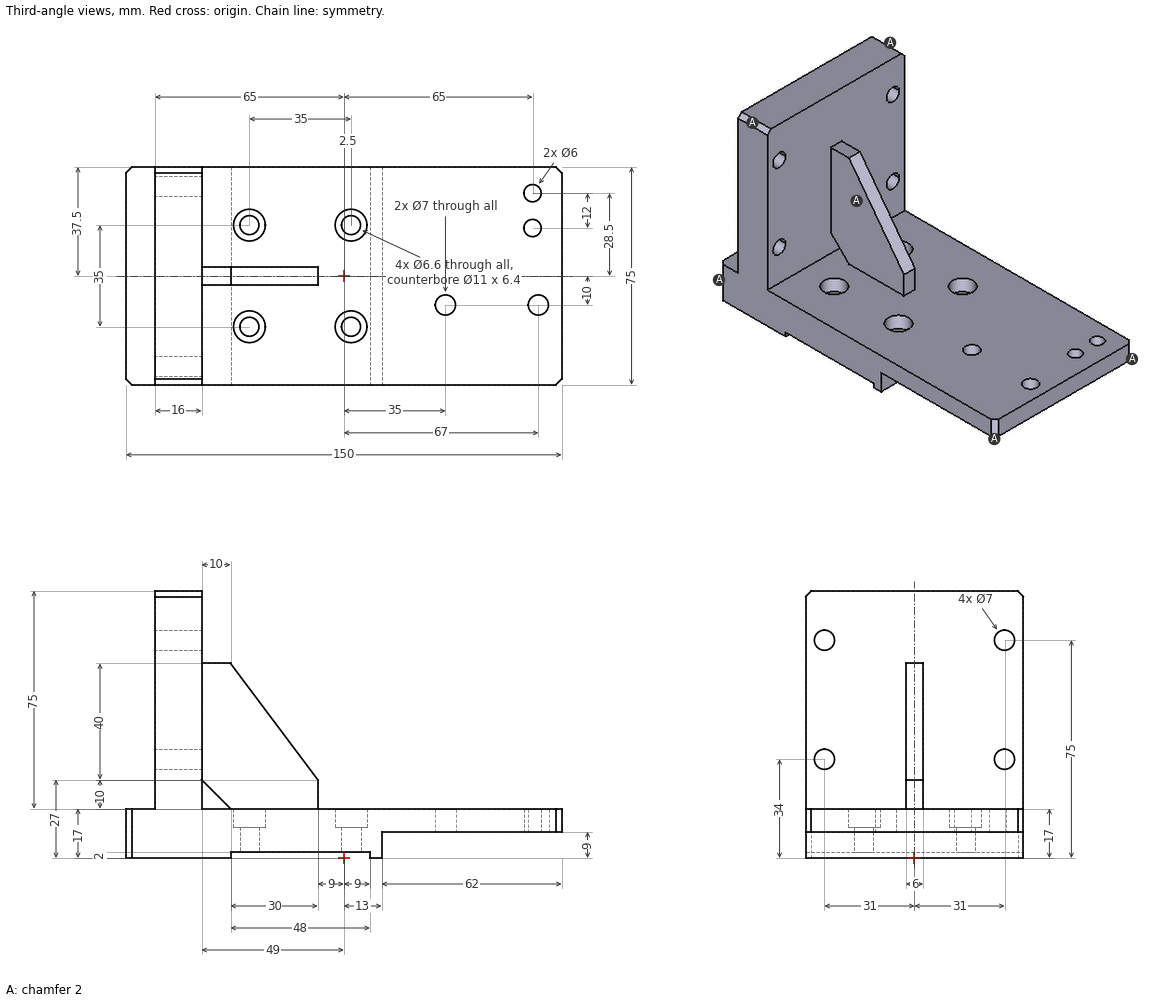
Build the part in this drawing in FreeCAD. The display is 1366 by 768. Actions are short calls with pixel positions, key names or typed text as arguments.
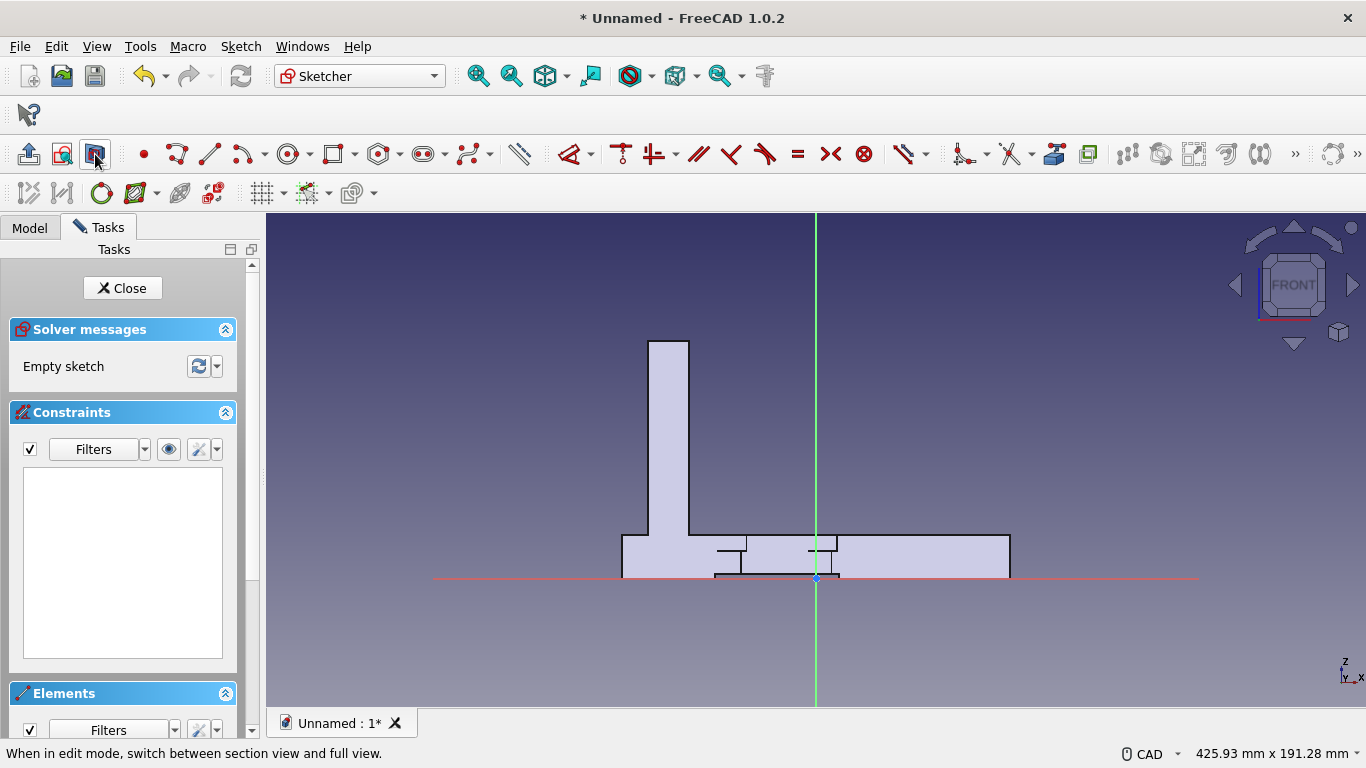
scroll(759, 532, up, 3)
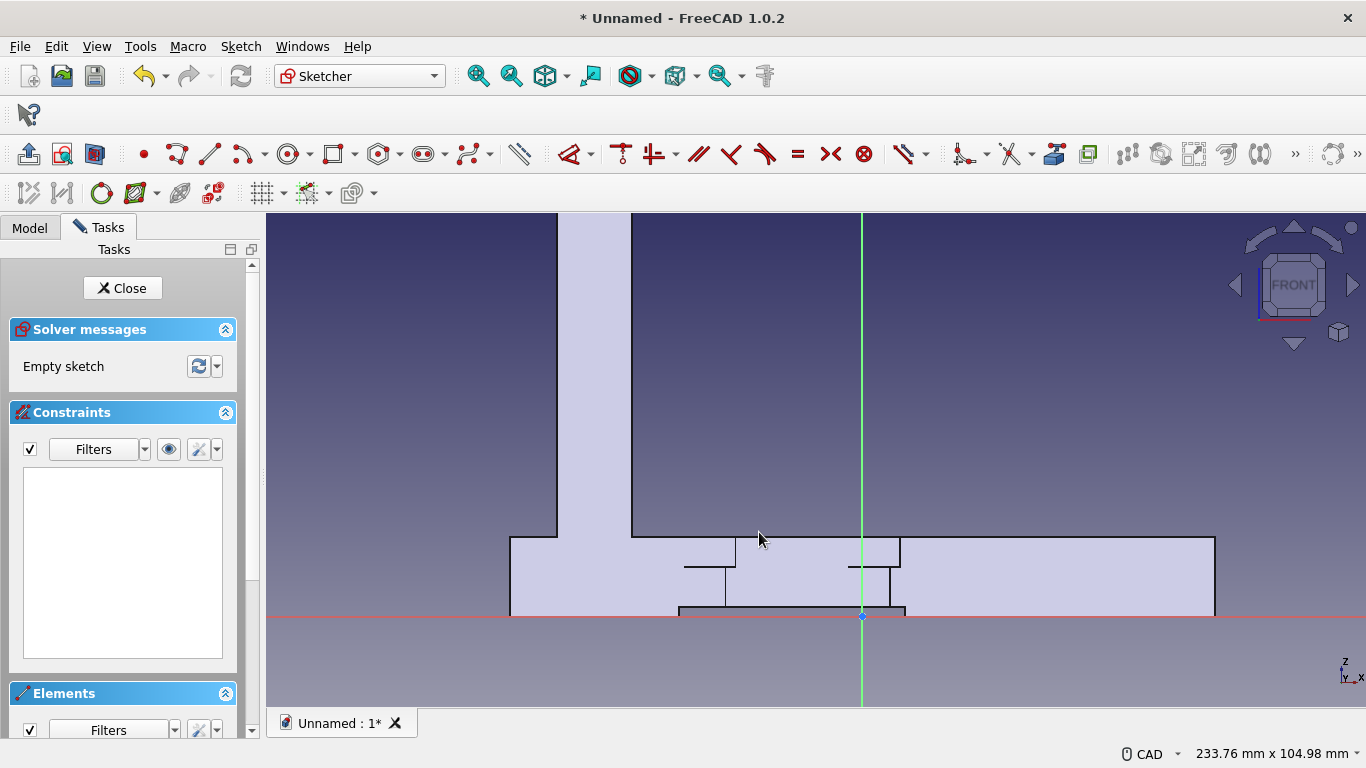
click(177, 154)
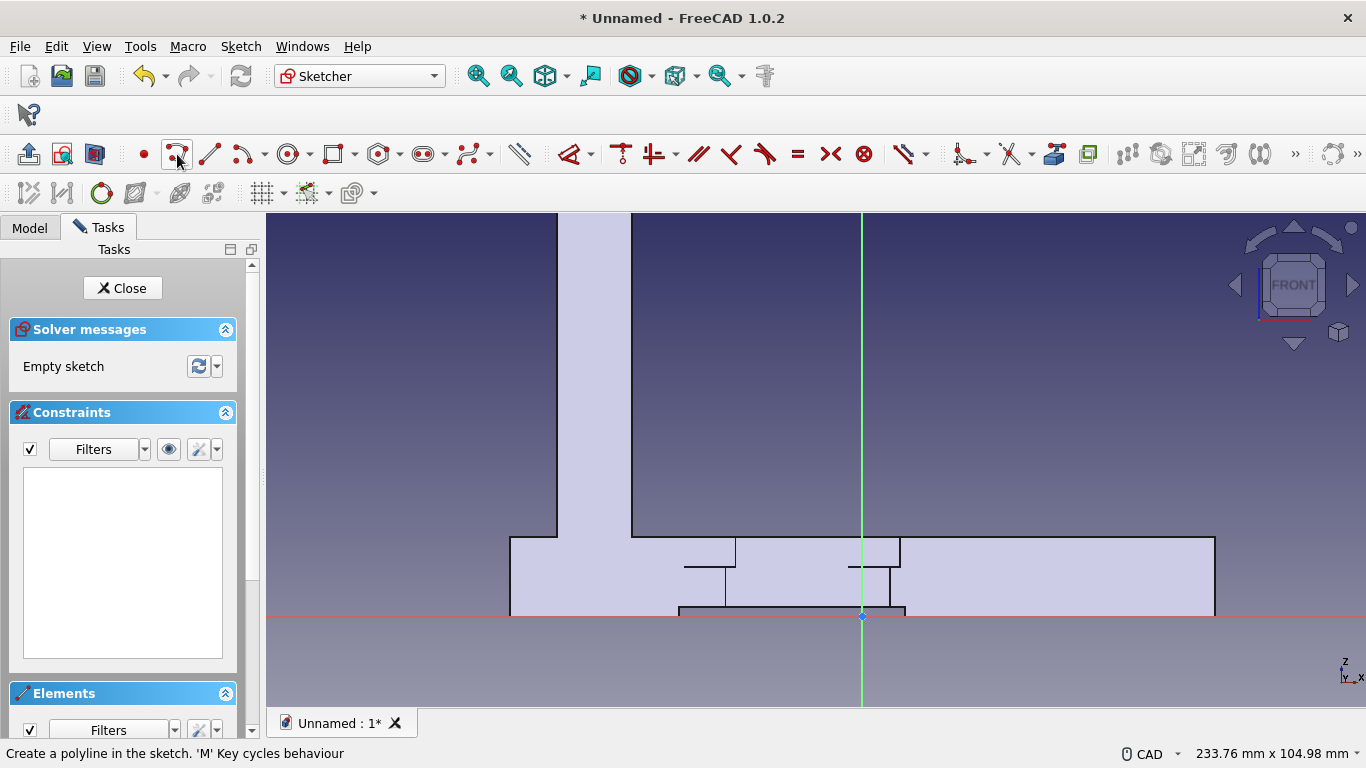
click(820, 537)
click(679, 537)
click(632, 490)
click(632, 301)
click(679, 301)
click(820, 490)
click(820, 538)
key(Escape)
key(Escape)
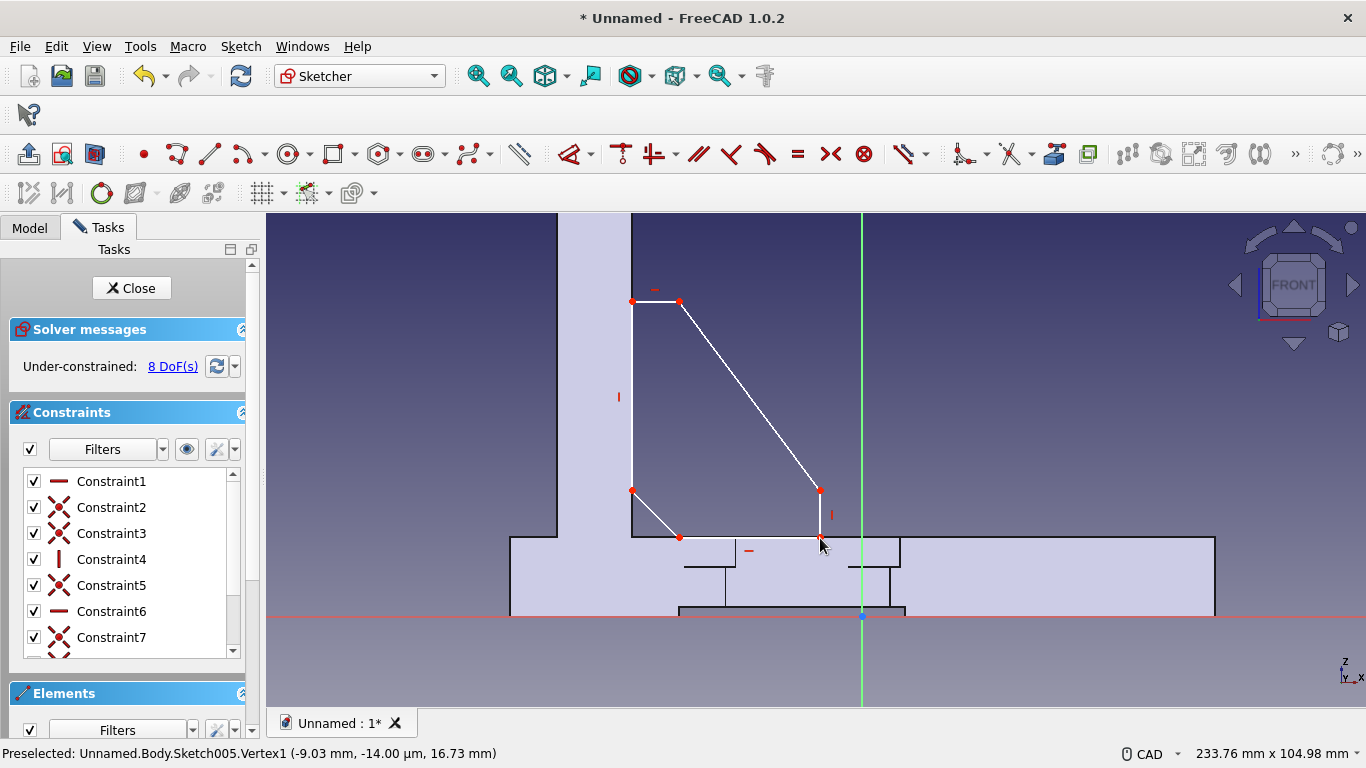
click(568, 154)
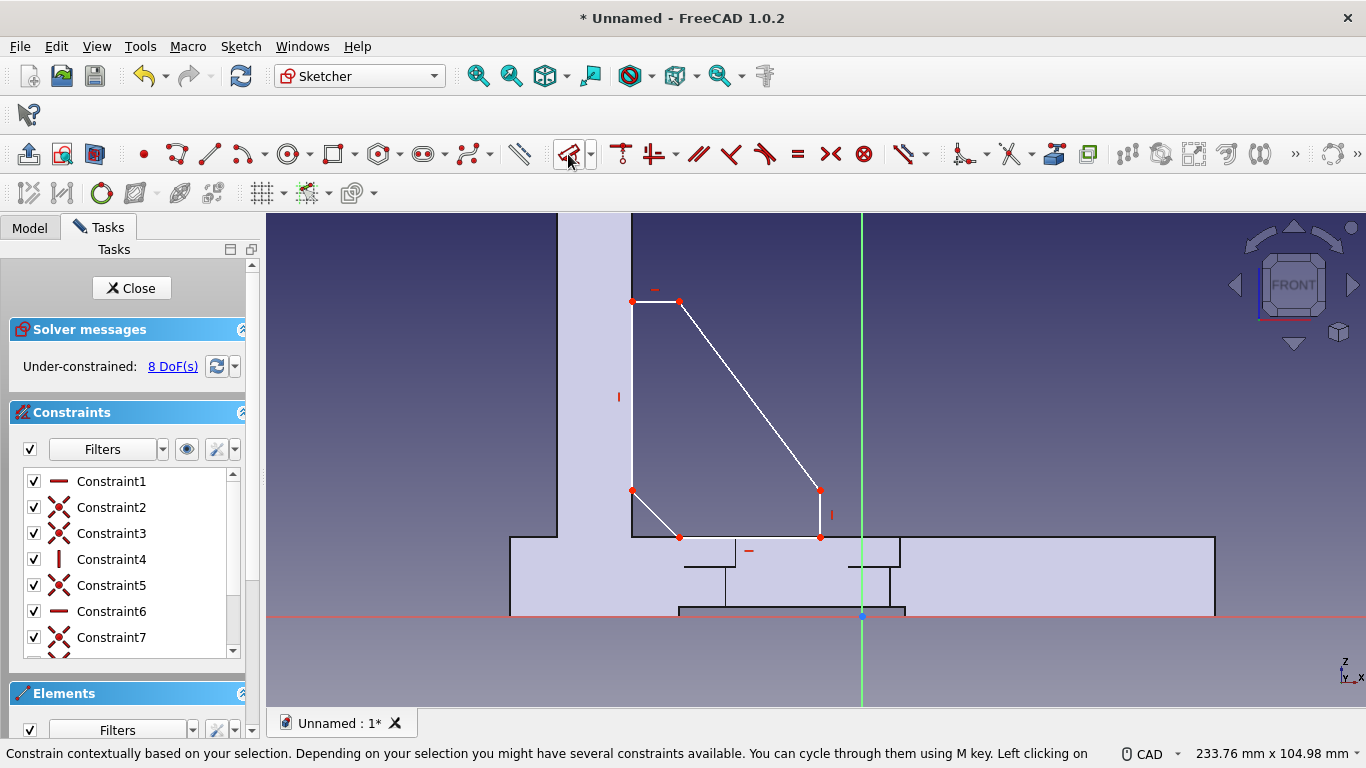
click(778, 538)
click(750, 572)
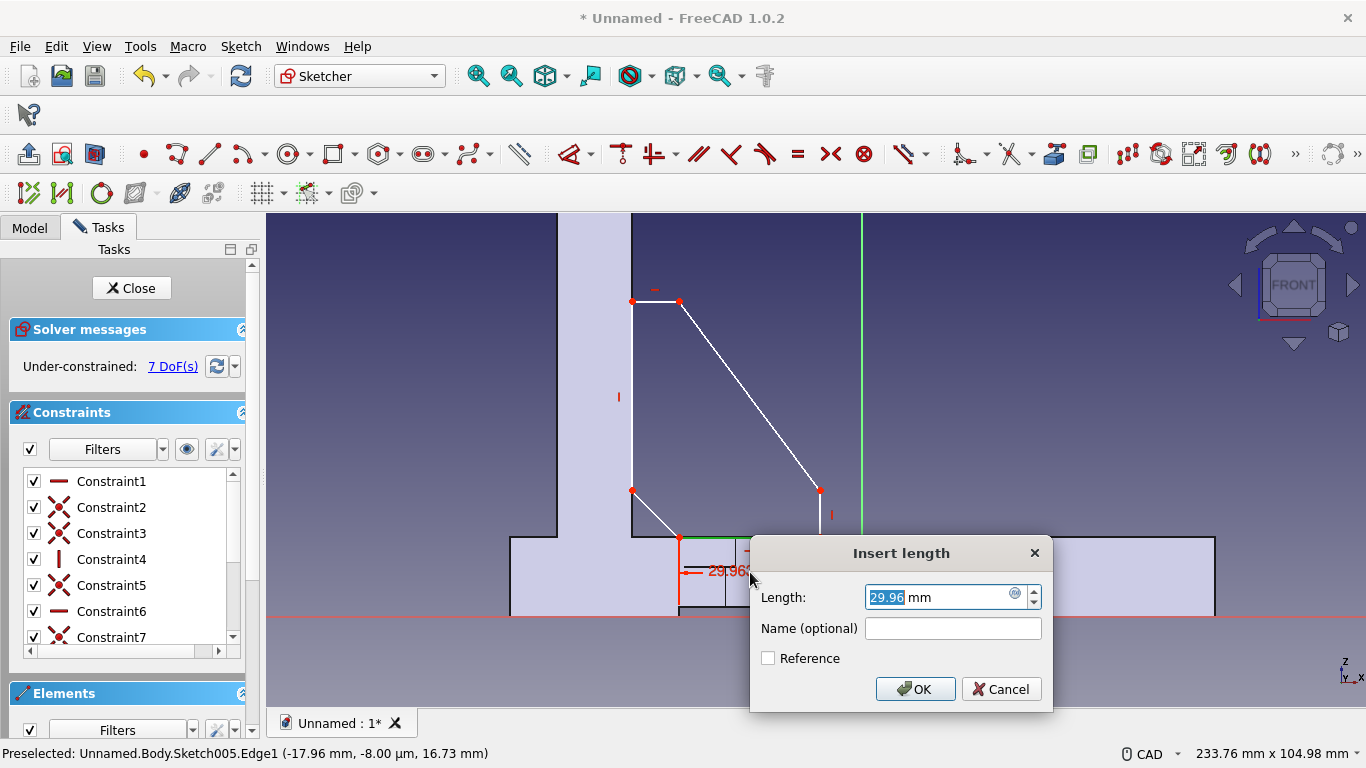
text(30)
key(Return)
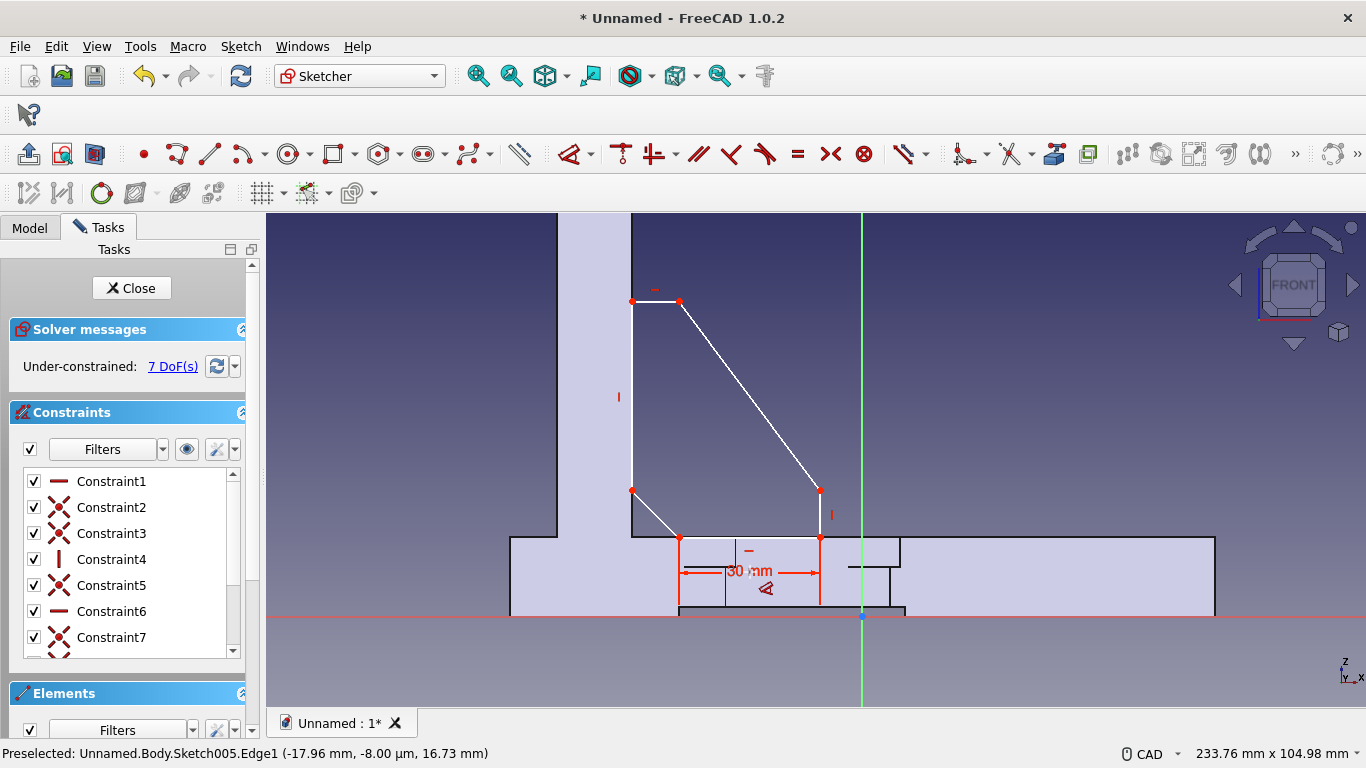
click(632, 434)
click(598, 397)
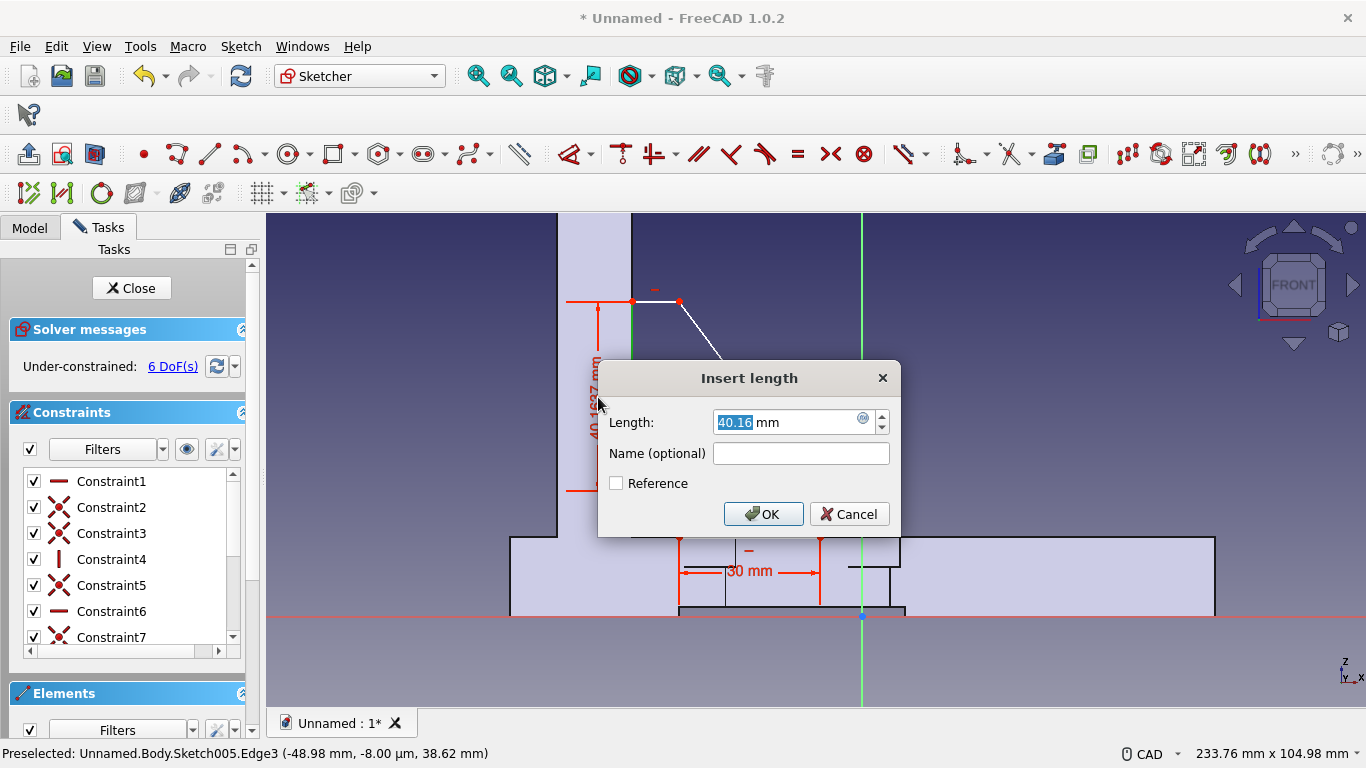
text(40)
key(Return)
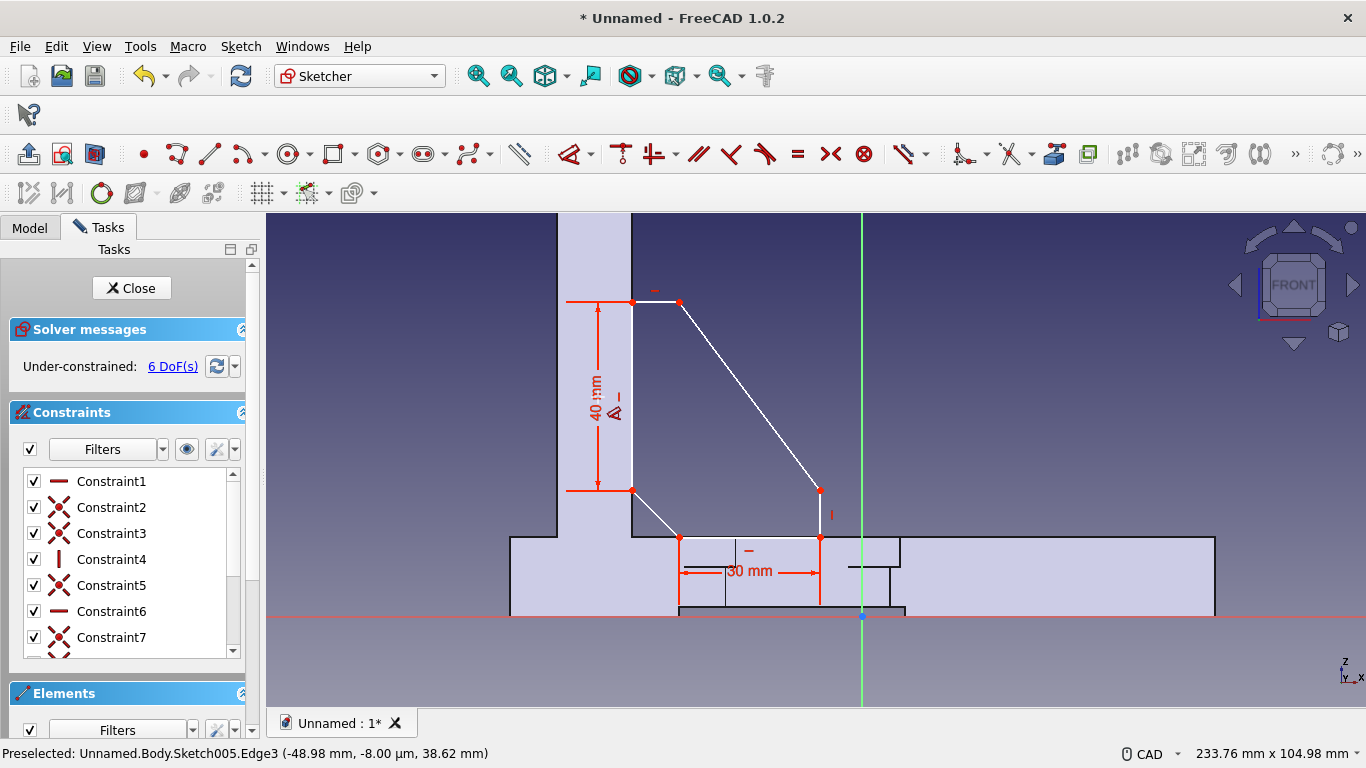
click(646, 302)
click(656, 268)